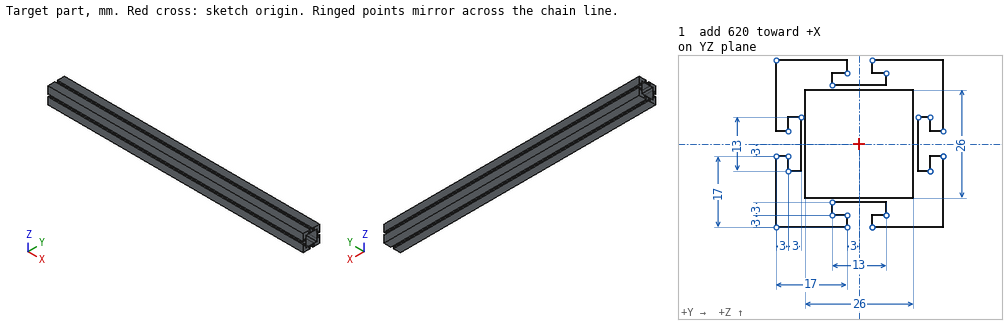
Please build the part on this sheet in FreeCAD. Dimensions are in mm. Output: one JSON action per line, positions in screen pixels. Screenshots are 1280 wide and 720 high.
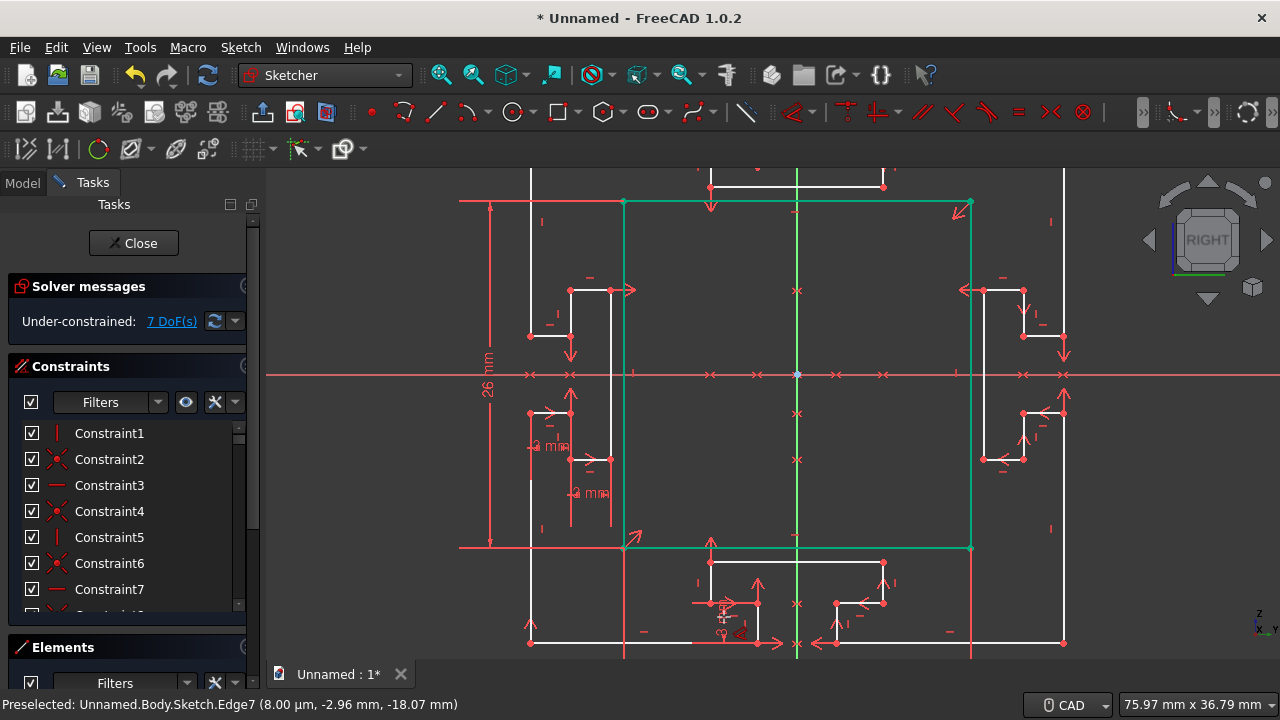
{"action": "left_click", "coordinate": [711, 591]}
{"action": "left_click", "coordinate": [677, 583]}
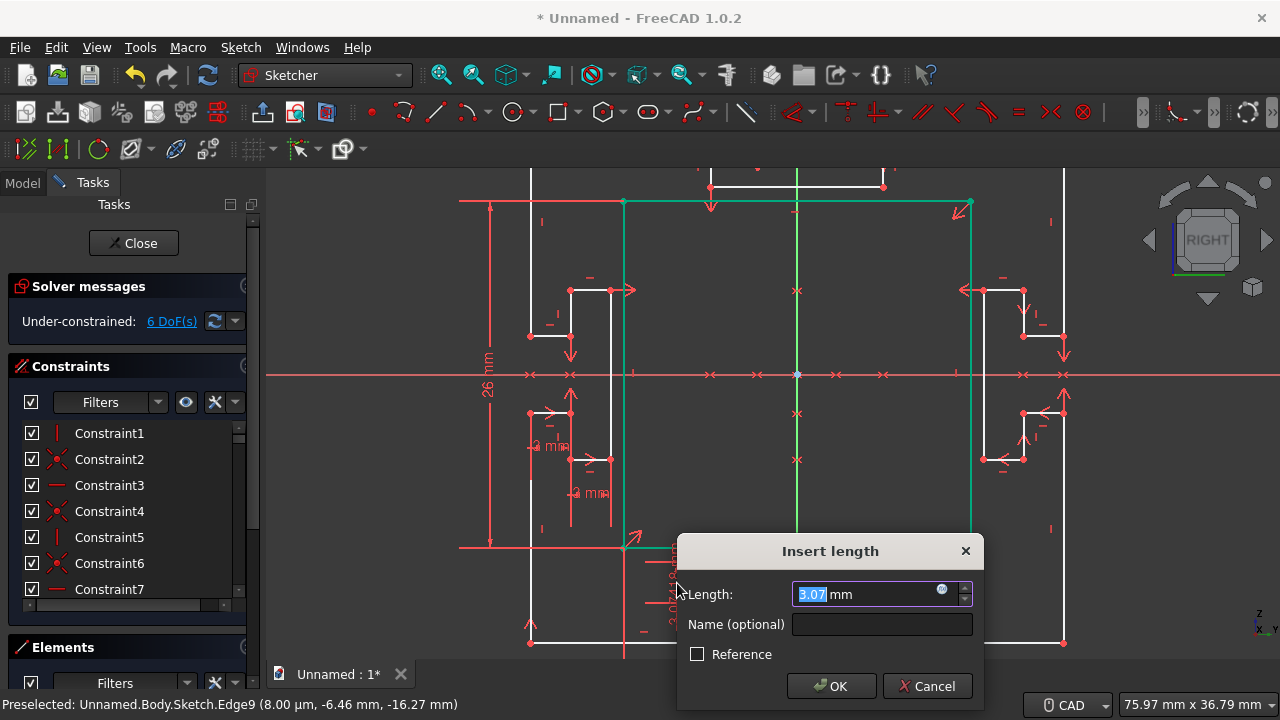
{"action": "type", "text": "3"}
{"action": "key", "text": "Return"}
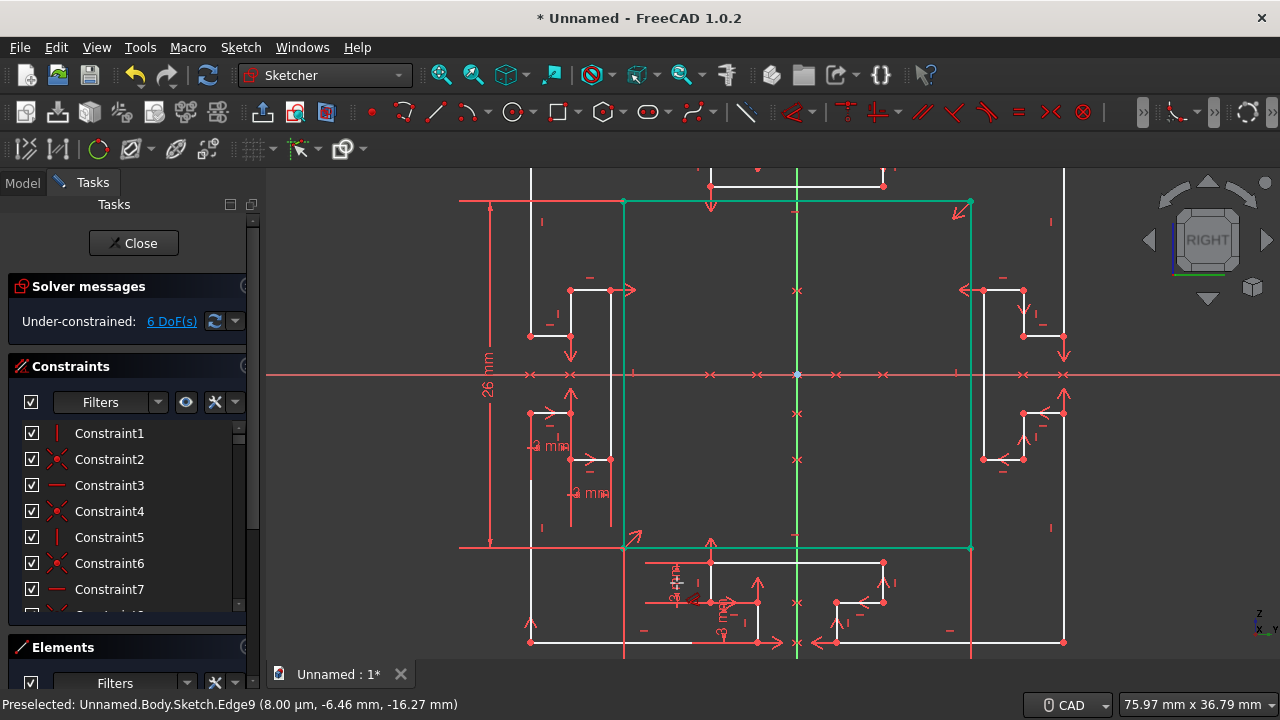
{"action": "left_click", "coordinate": [611, 341]}
{"action": "left_click", "coordinate": [645, 336]}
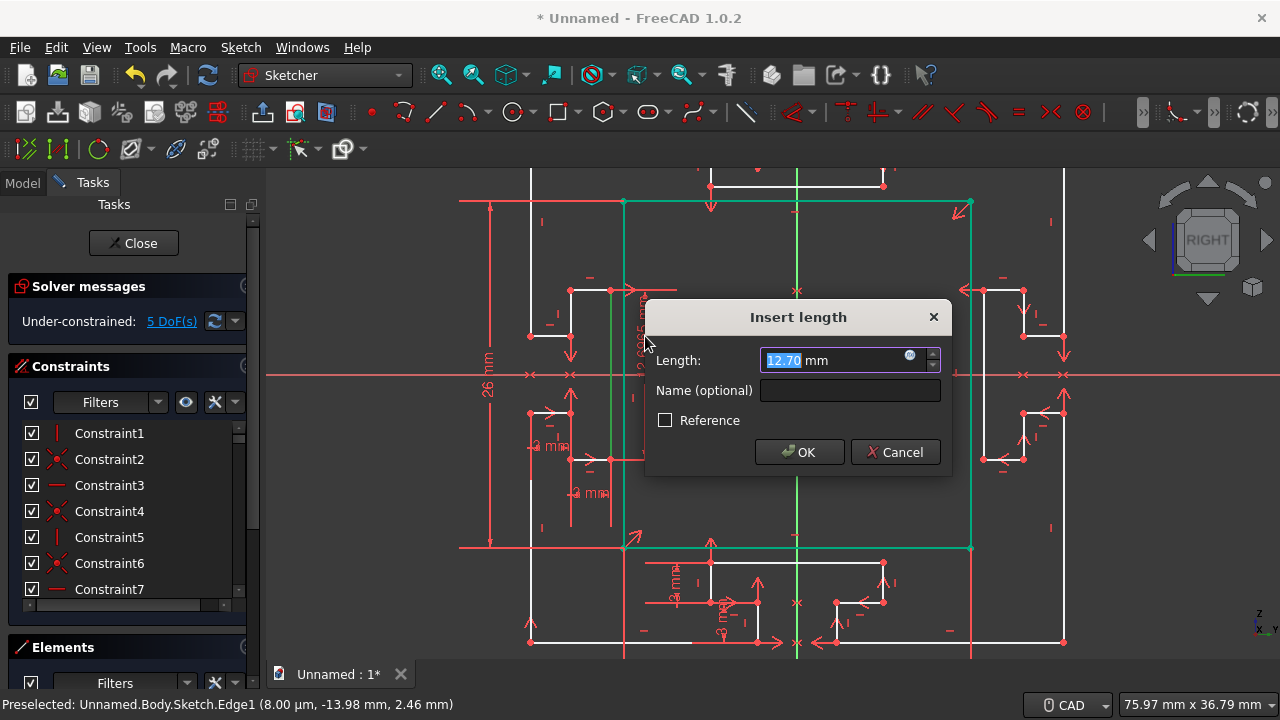
{"action": "type", "text": "13"}
{"action": "key", "text": "Return"}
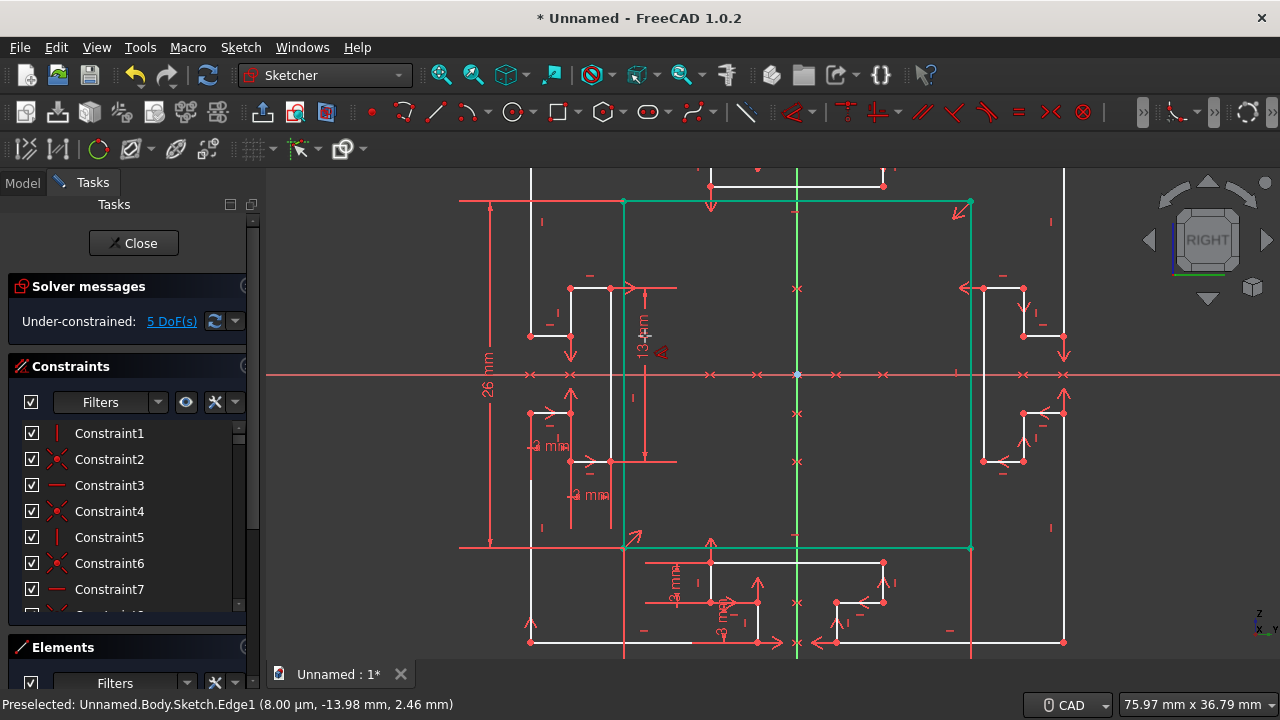
{"action": "left_click", "coordinate": [531, 482]}
{"action": "left_click", "coordinate": [497, 522]}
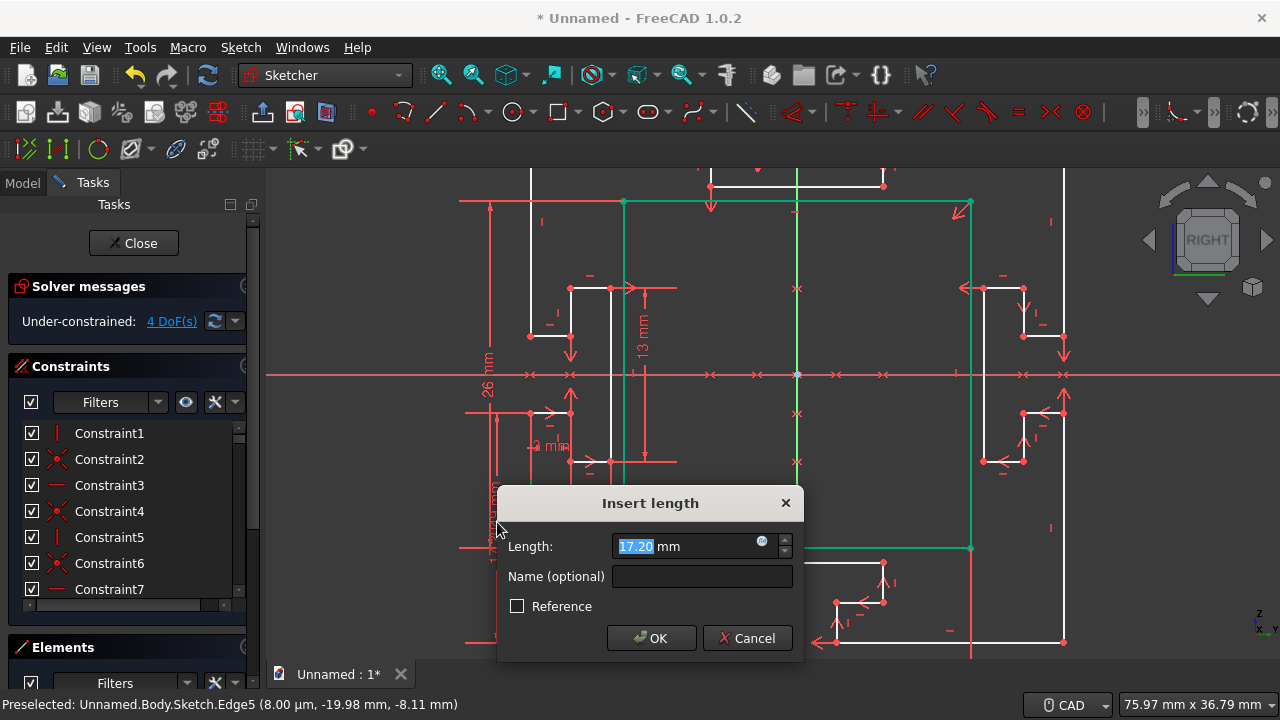
{"action": "type", "text": "17"}
{"action": "key", "text": "Return"}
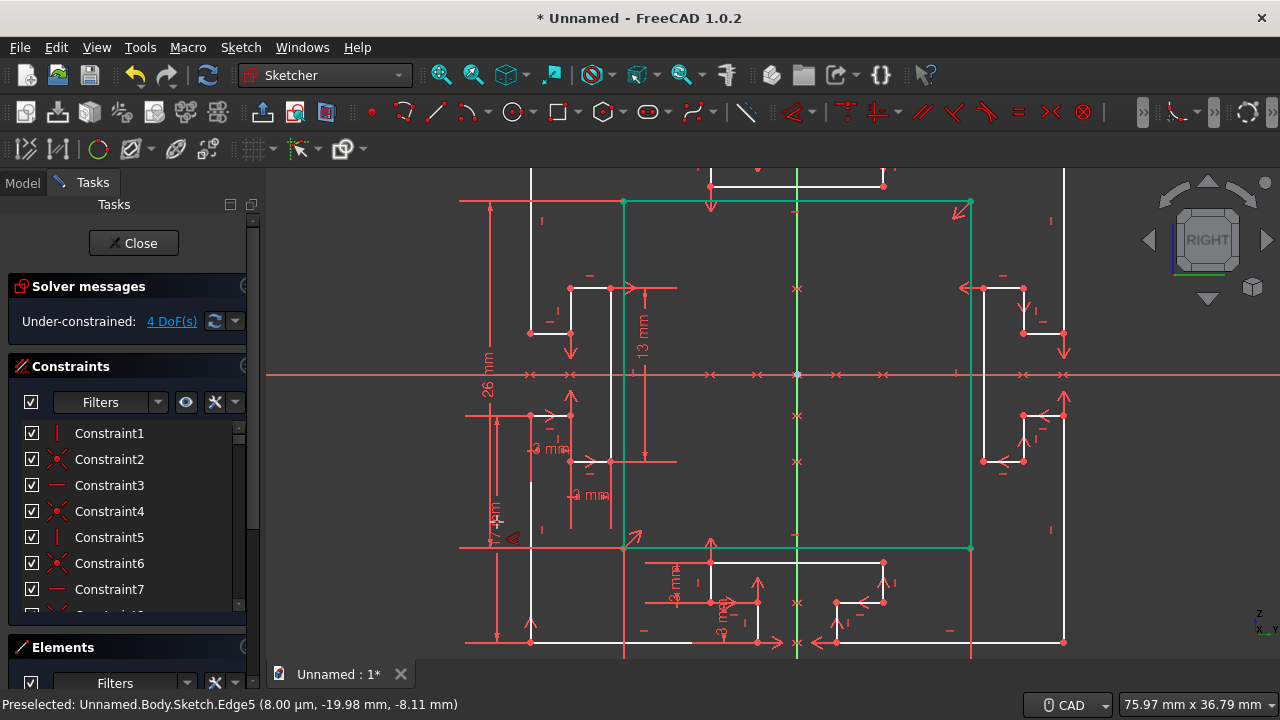
{"action": "scroll", "coordinate": [592, 461], "scroll_direction": "down", "scroll_amount": 3}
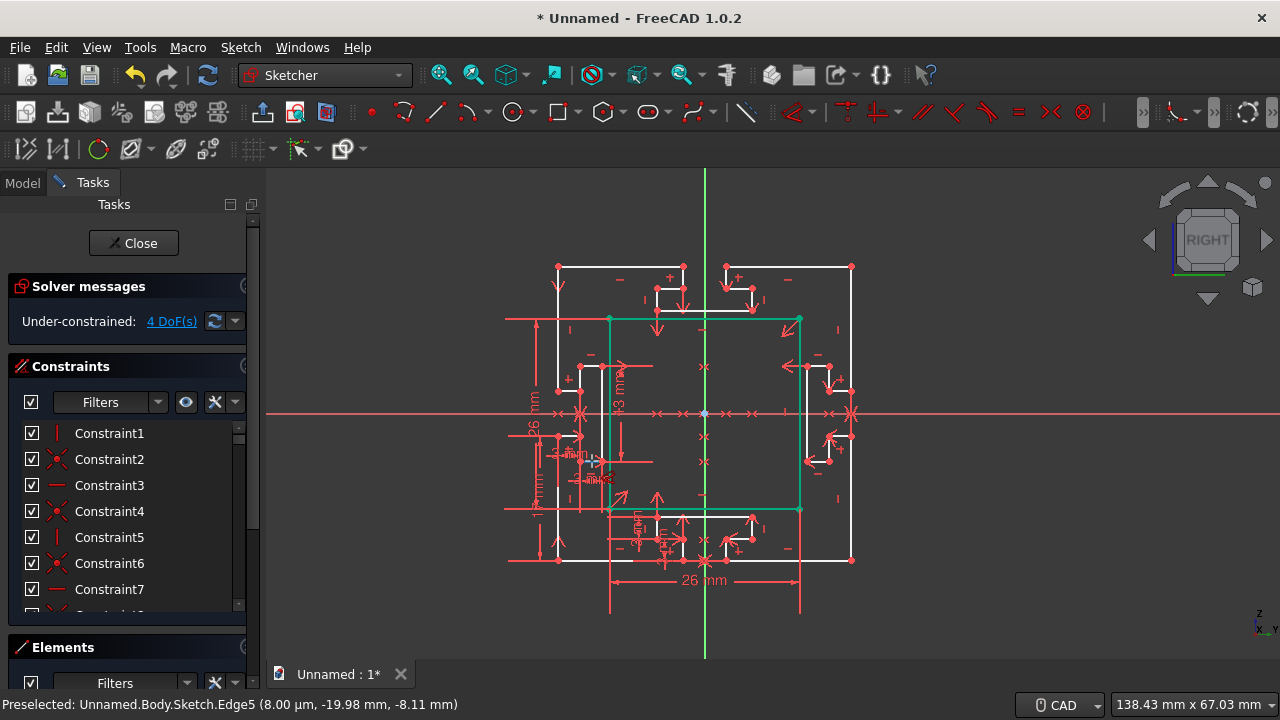
{"action": "left_click", "coordinate": [596, 561]}
{"action": "left_click", "coordinate": [621, 595]}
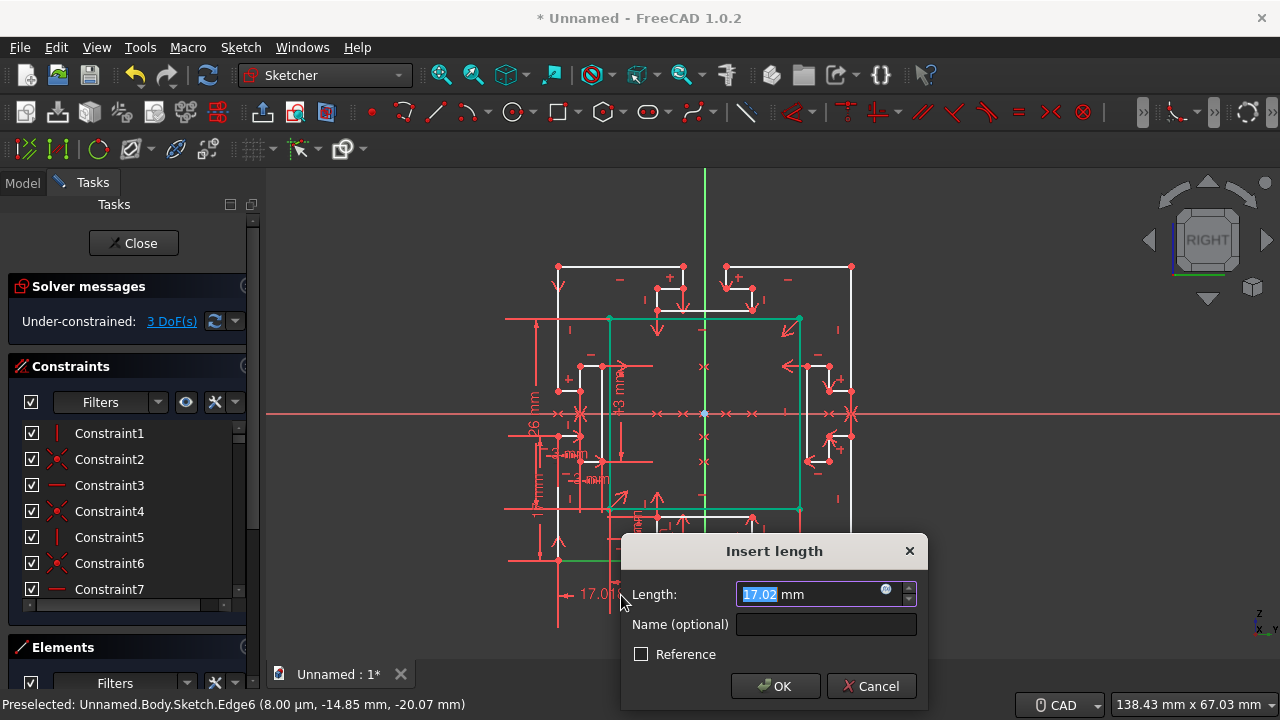
{"action": "type", "text": "17"}
{"action": "key", "text": "Return"}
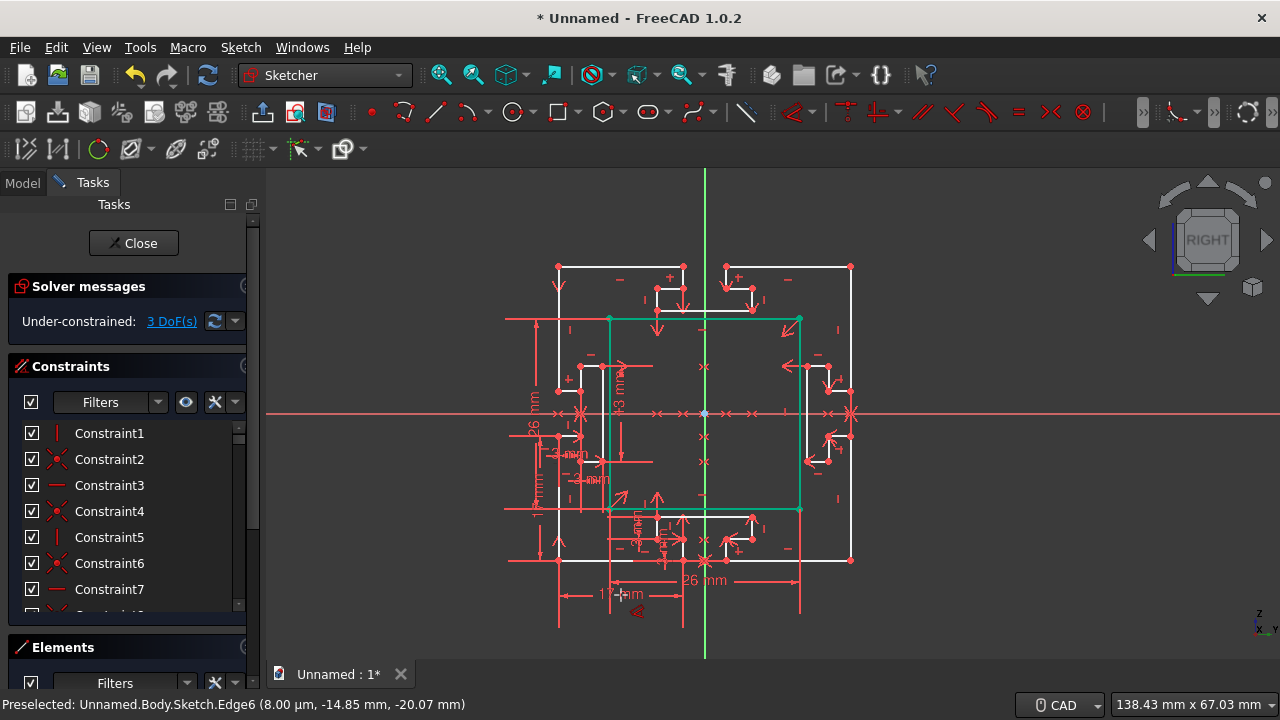
{"action": "scroll", "coordinate": [686, 517], "scroll_direction": "up", "scroll_amount": 3}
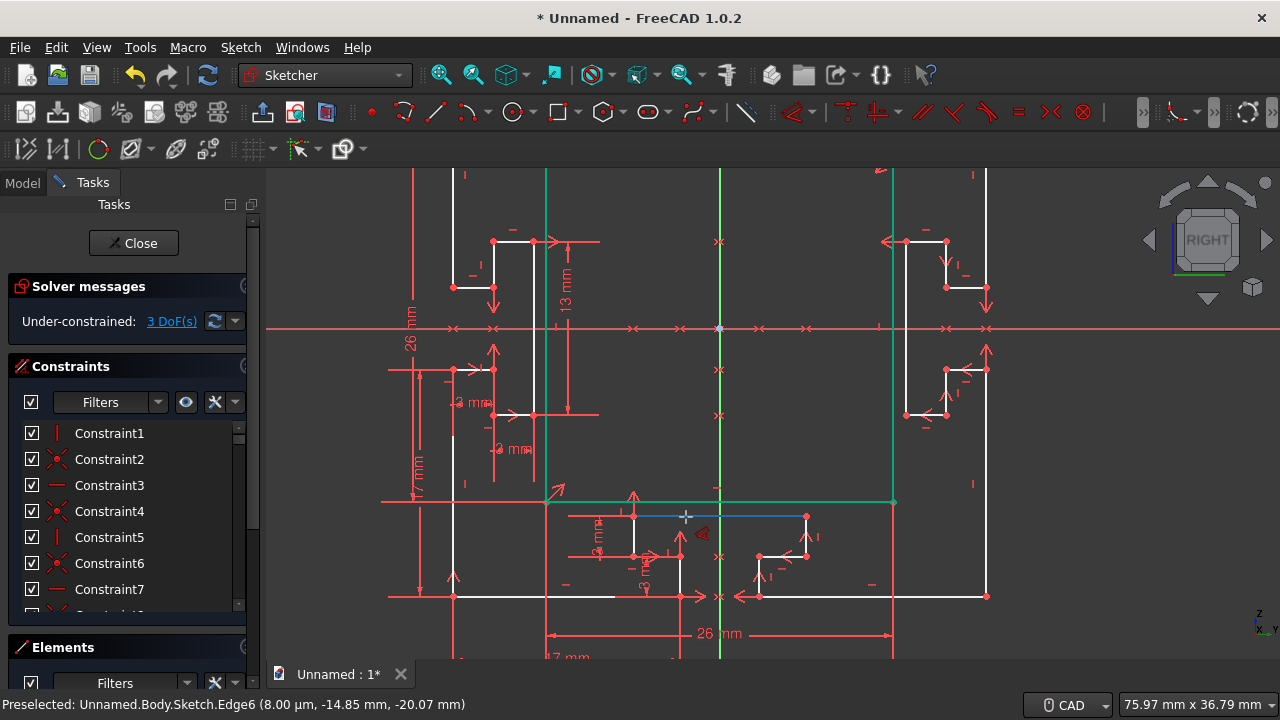
{"action": "left_click", "coordinate": [685, 516]}
{"action": "left_click", "coordinate": [680, 482]}